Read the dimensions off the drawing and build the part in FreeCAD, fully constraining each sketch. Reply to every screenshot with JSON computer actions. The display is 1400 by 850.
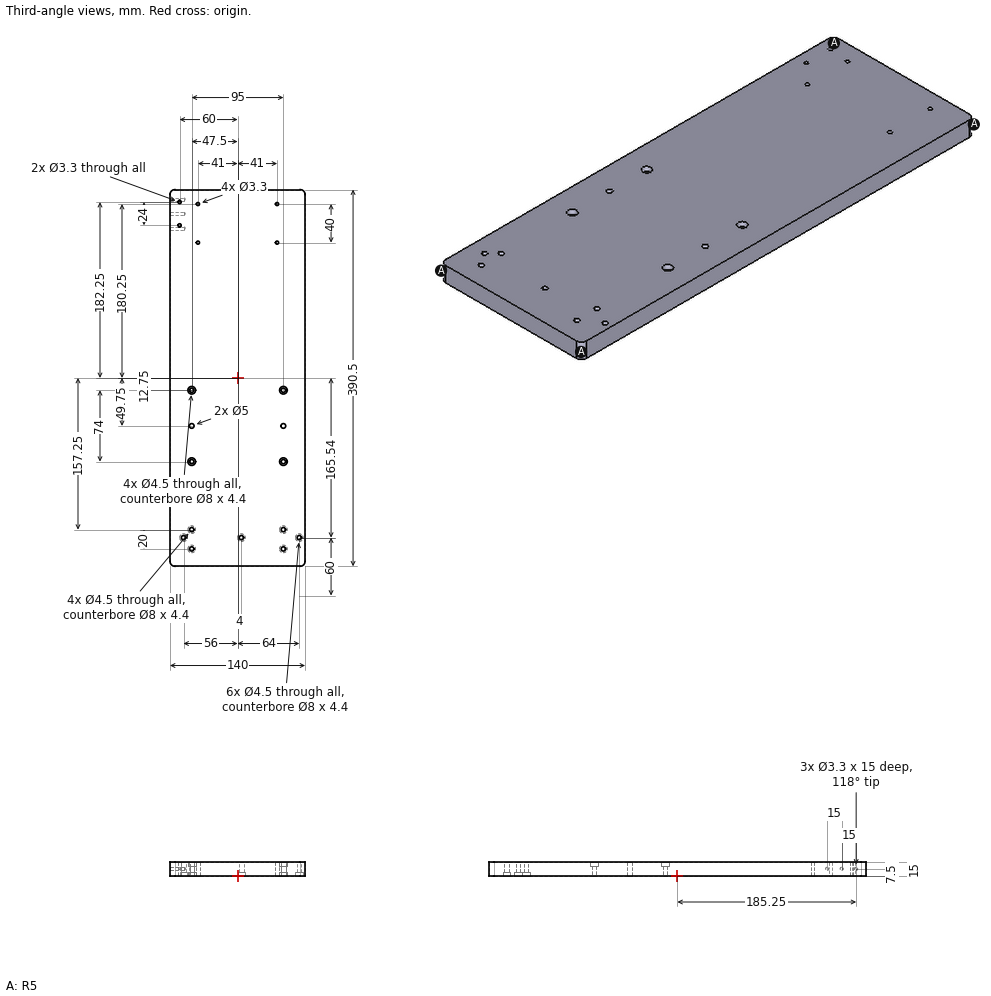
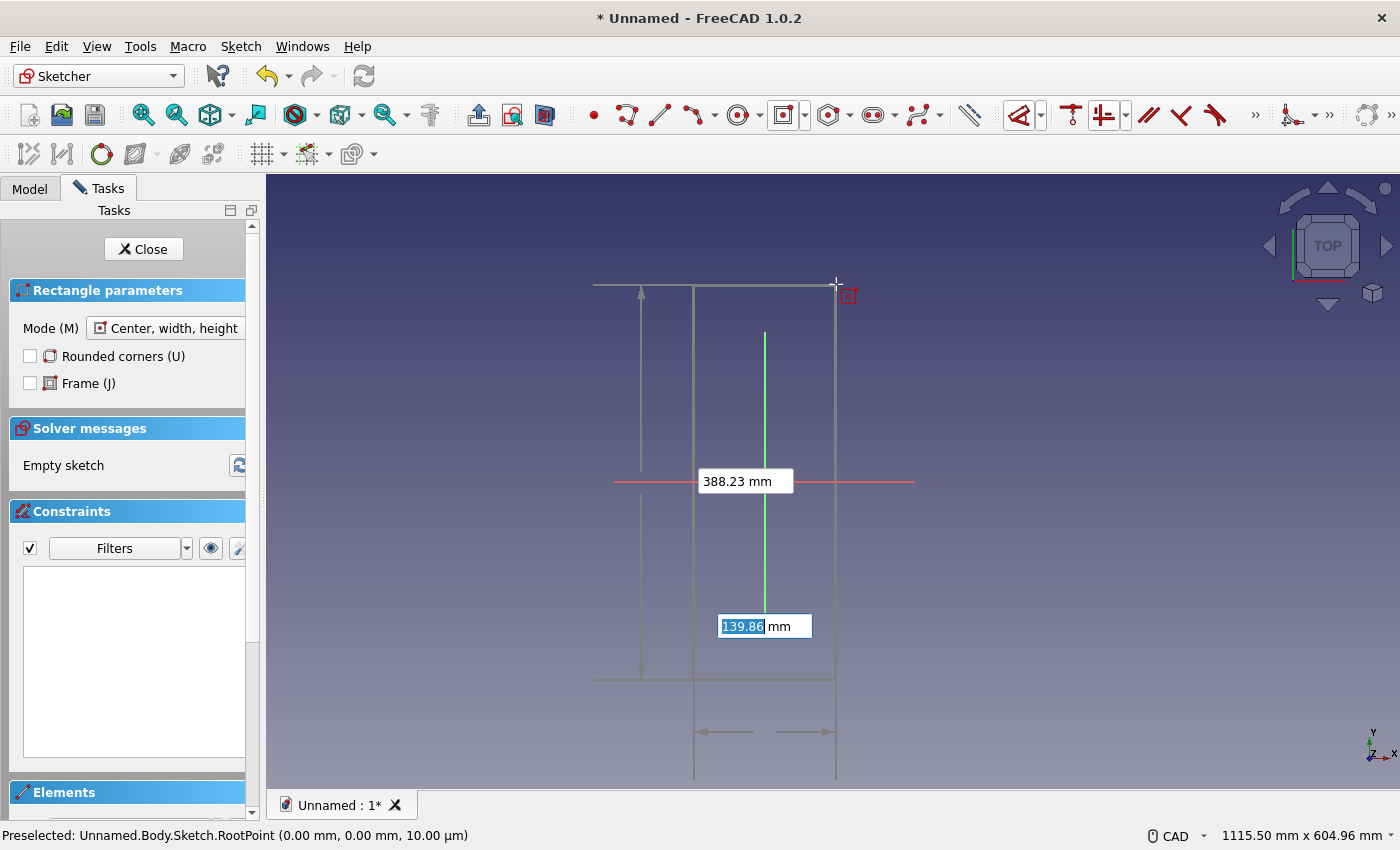
{"action": "type", "text": "140"}
{"action": "key", "text": "Tab"}
{"action": "type", "text": "390.5"}
{"action": "key", "text": "Return"}
{"action": "key", "text": "Escape"}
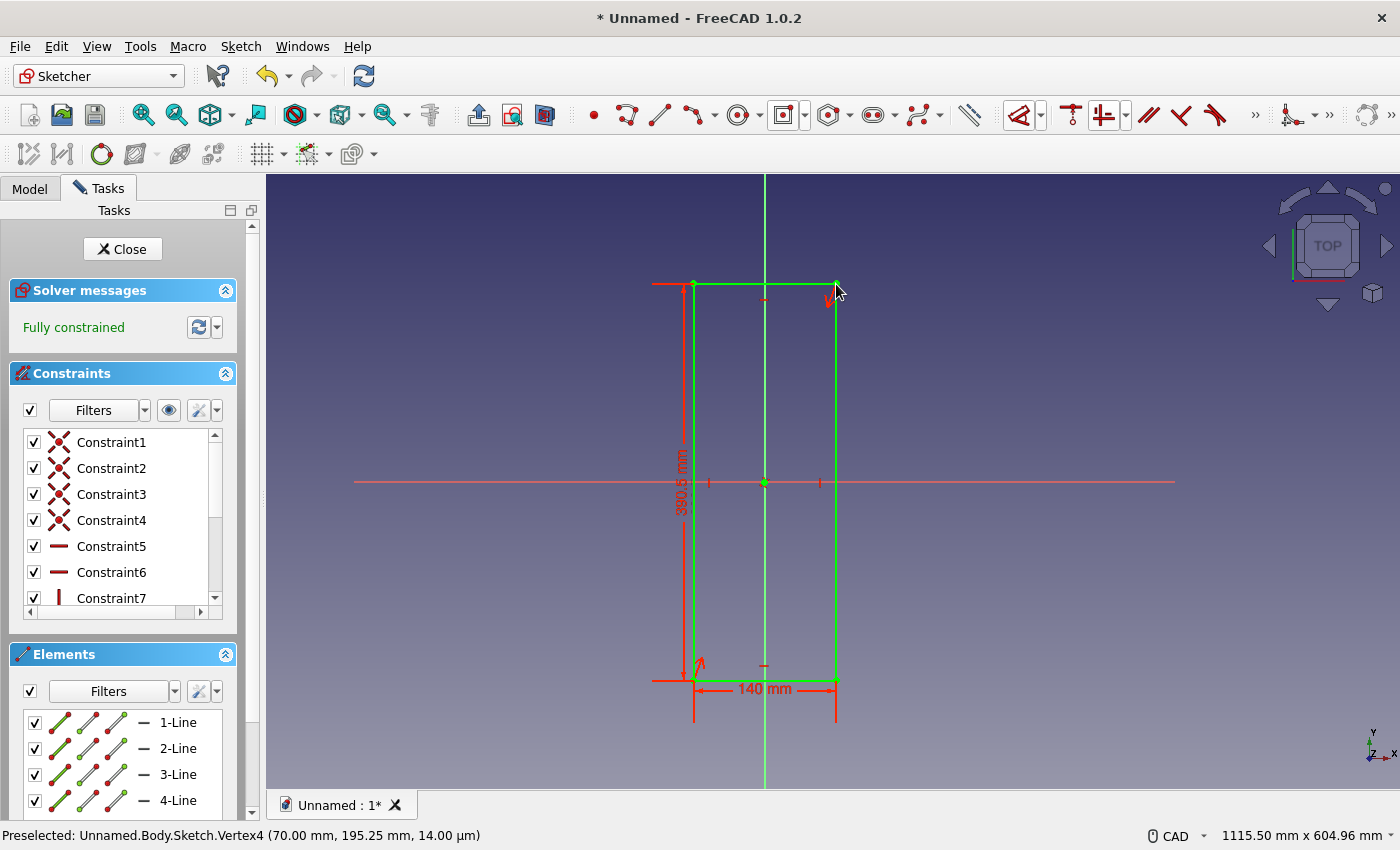
{"action": "left_click", "coordinate": [123, 249]}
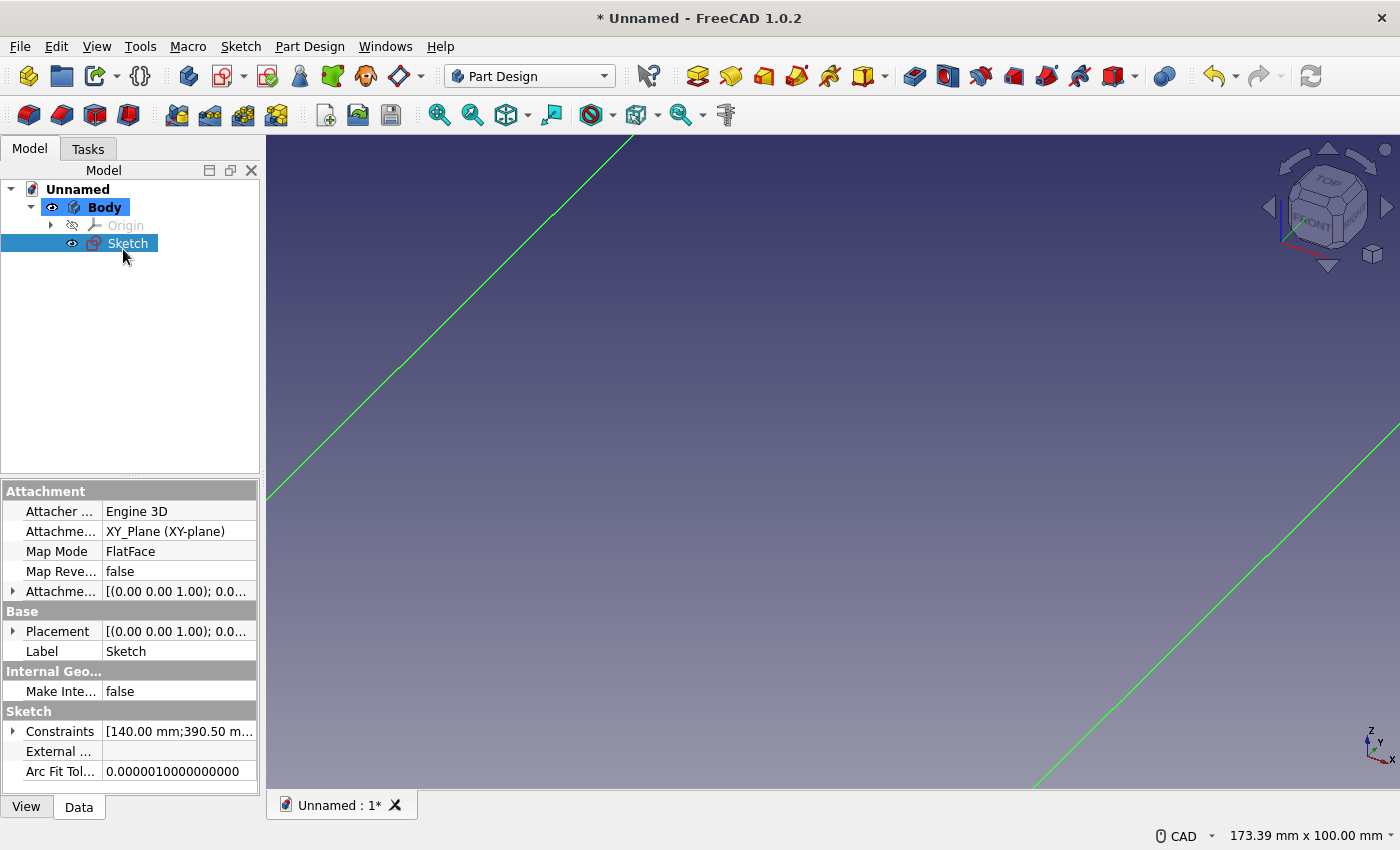
{"action": "left_click", "coordinate": [698, 76]}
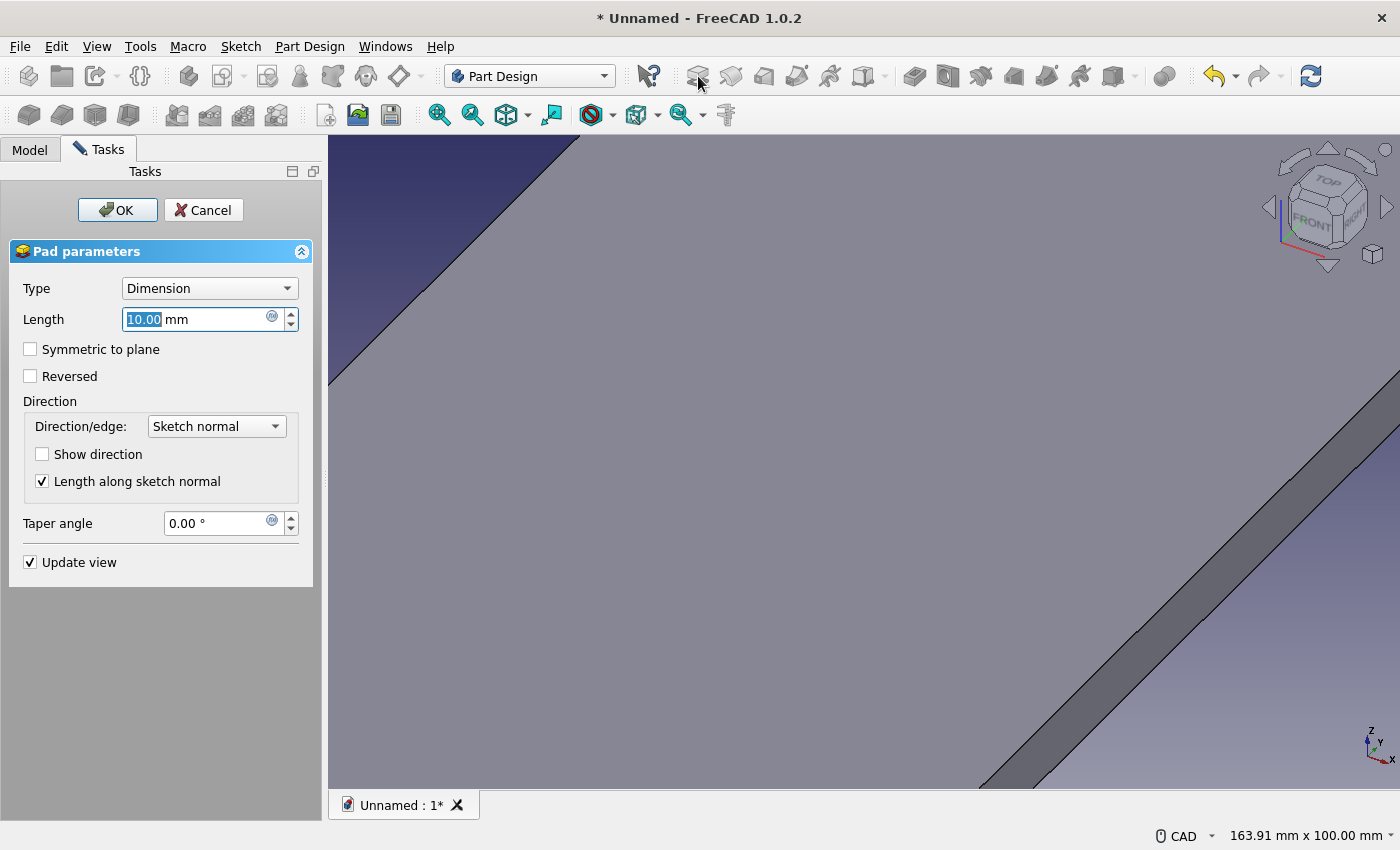
{"action": "type", "text": "15"}
{"action": "key", "text": "Tab"}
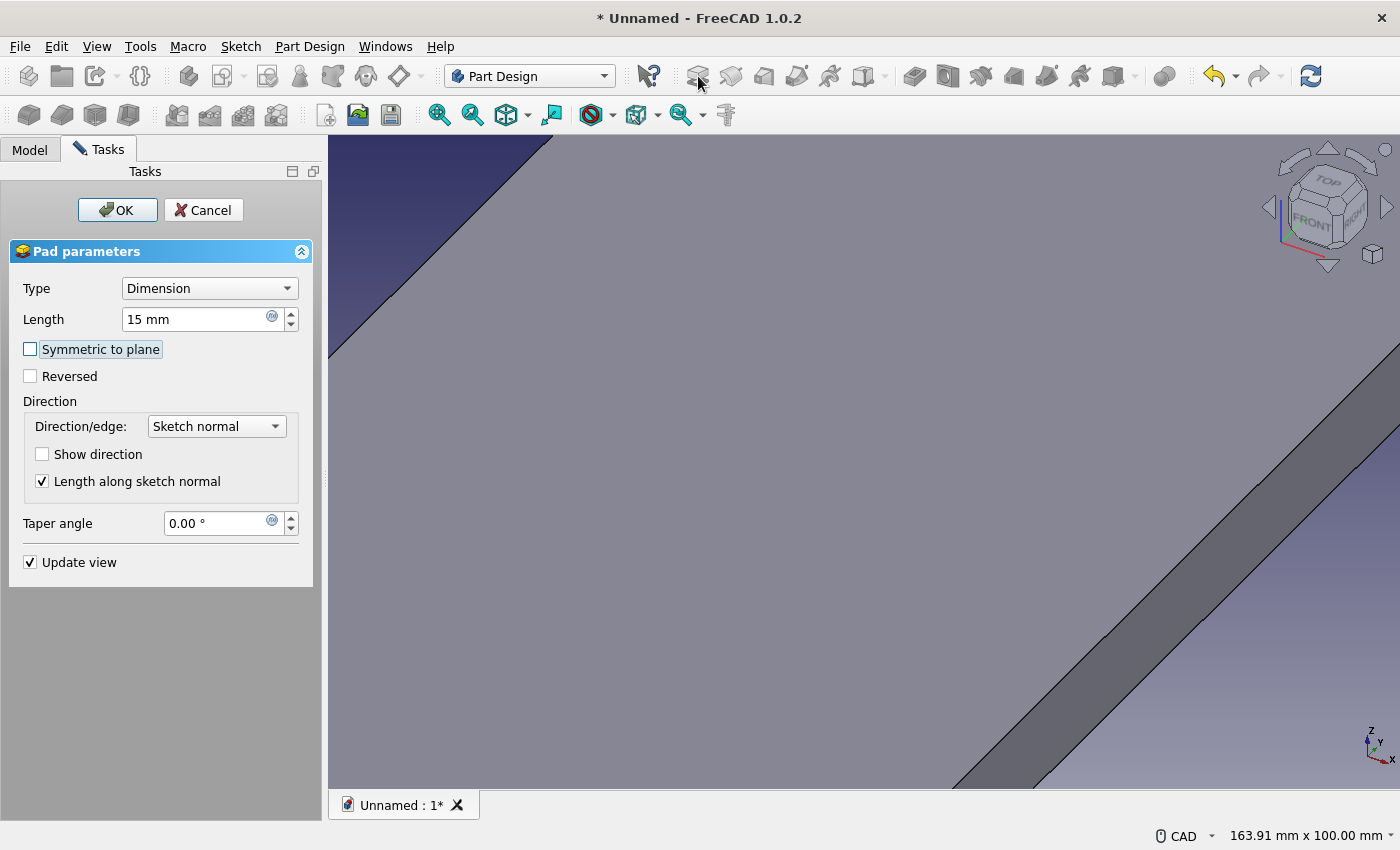
{"action": "left_click", "coordinate": [118, 210]}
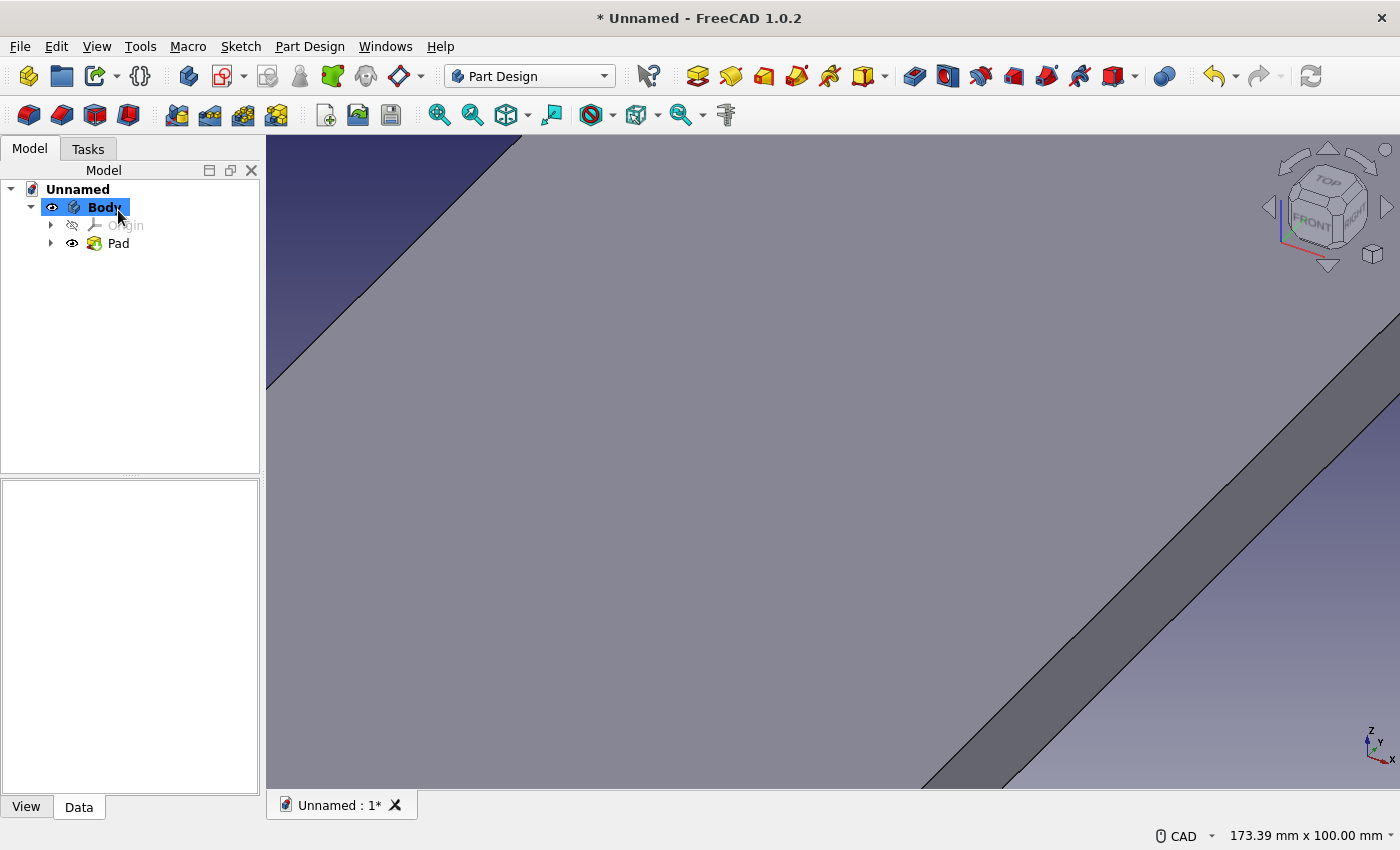
{"action": "left_click", "coordinate": [440, 116]}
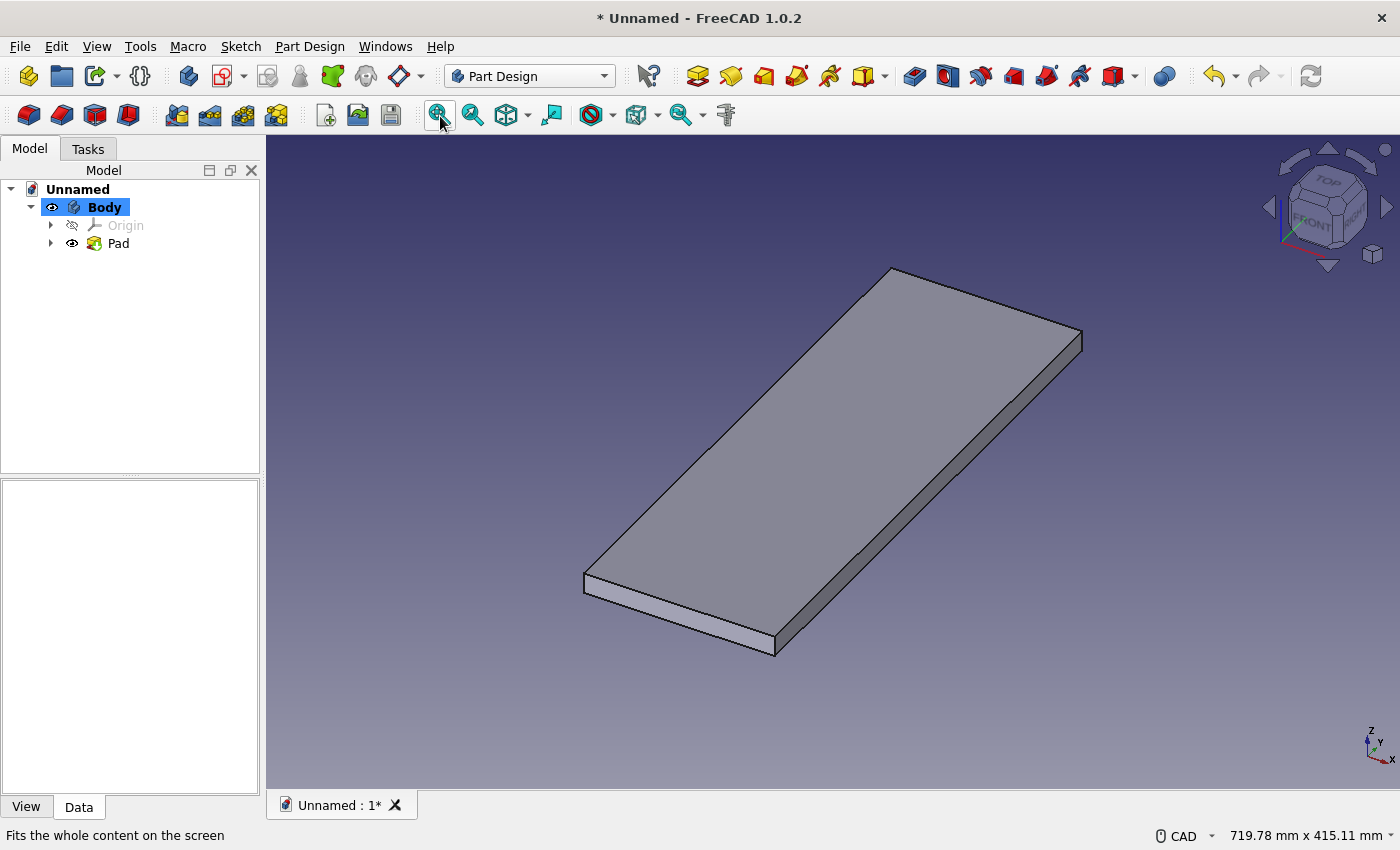
{"action": "left_click", "coordinate": [921, 364]}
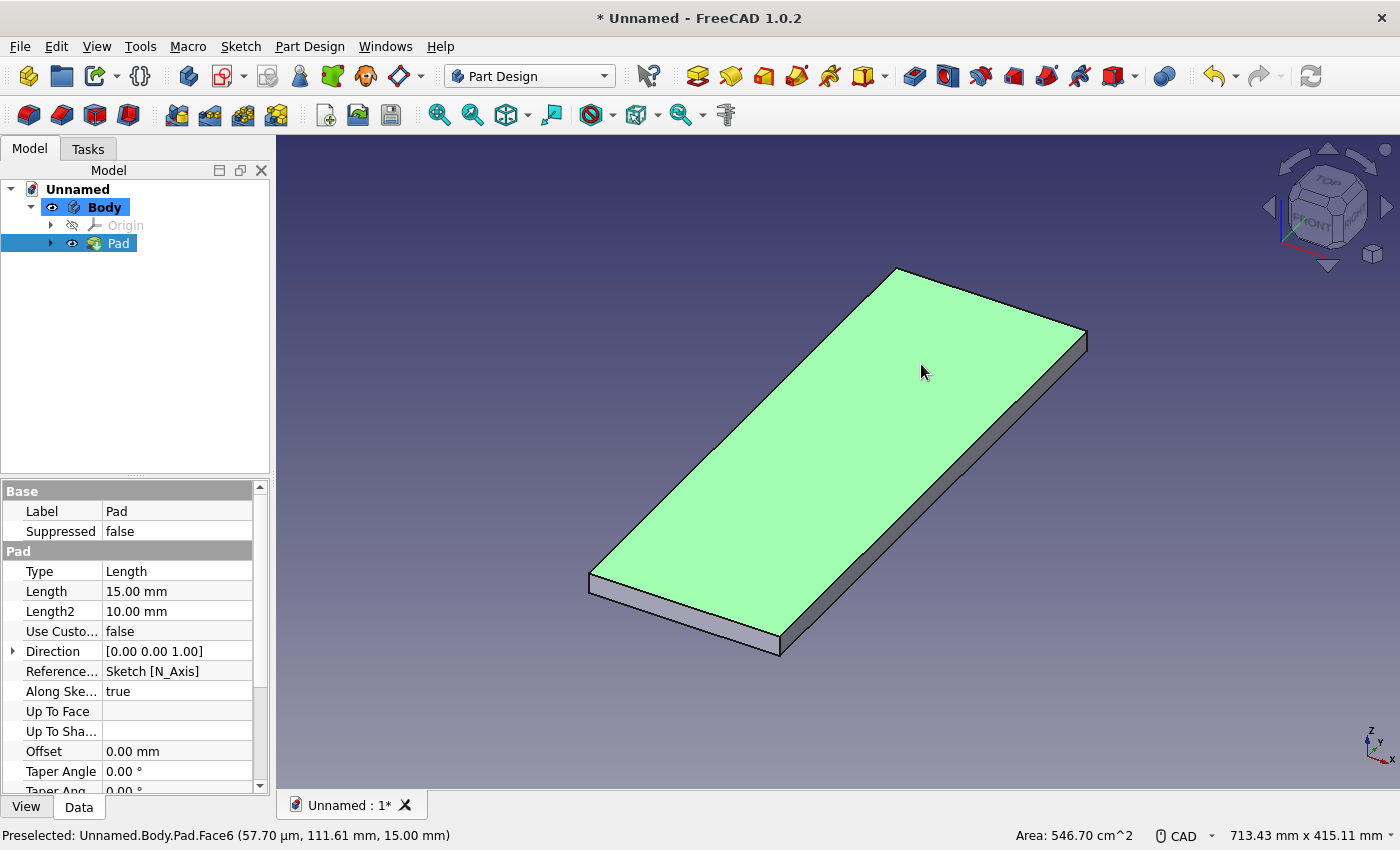
{"action": "left_click", "coordinate": [222, 76]}